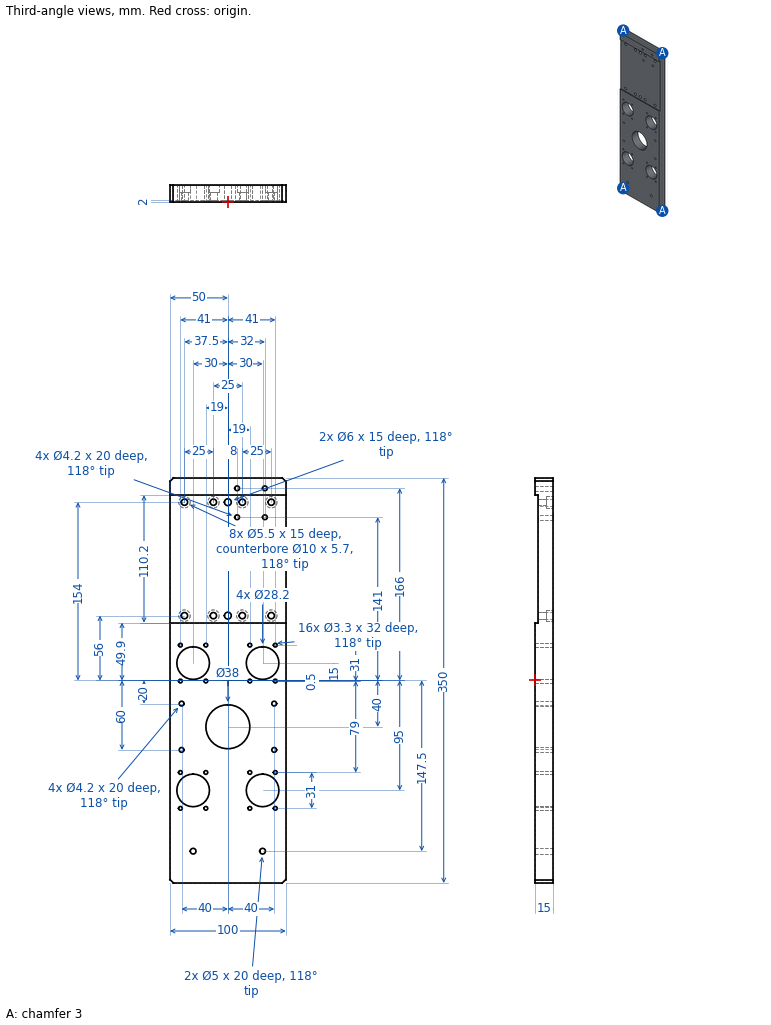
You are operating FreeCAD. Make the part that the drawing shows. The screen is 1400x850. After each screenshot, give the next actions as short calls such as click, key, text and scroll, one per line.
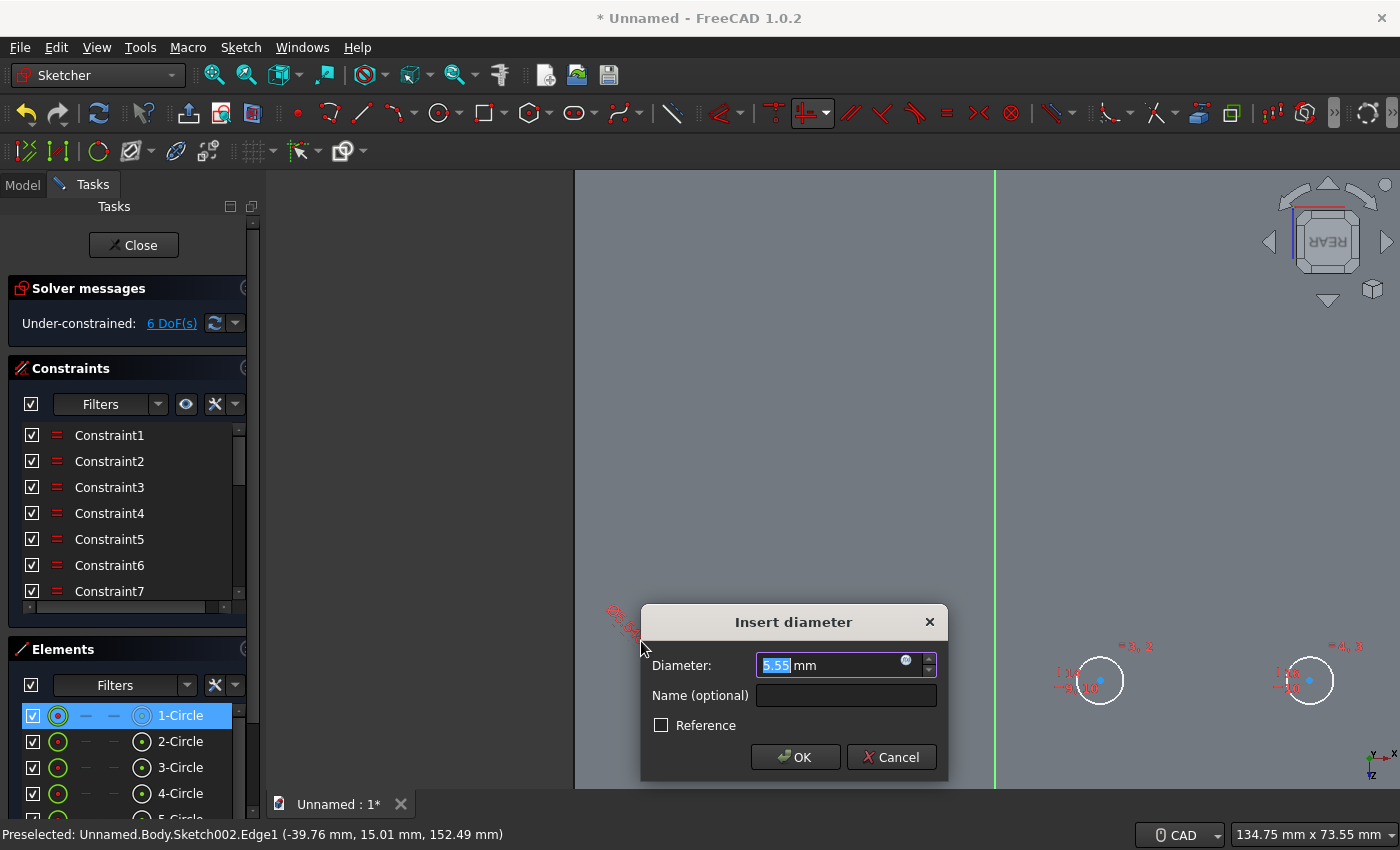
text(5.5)
key(Return)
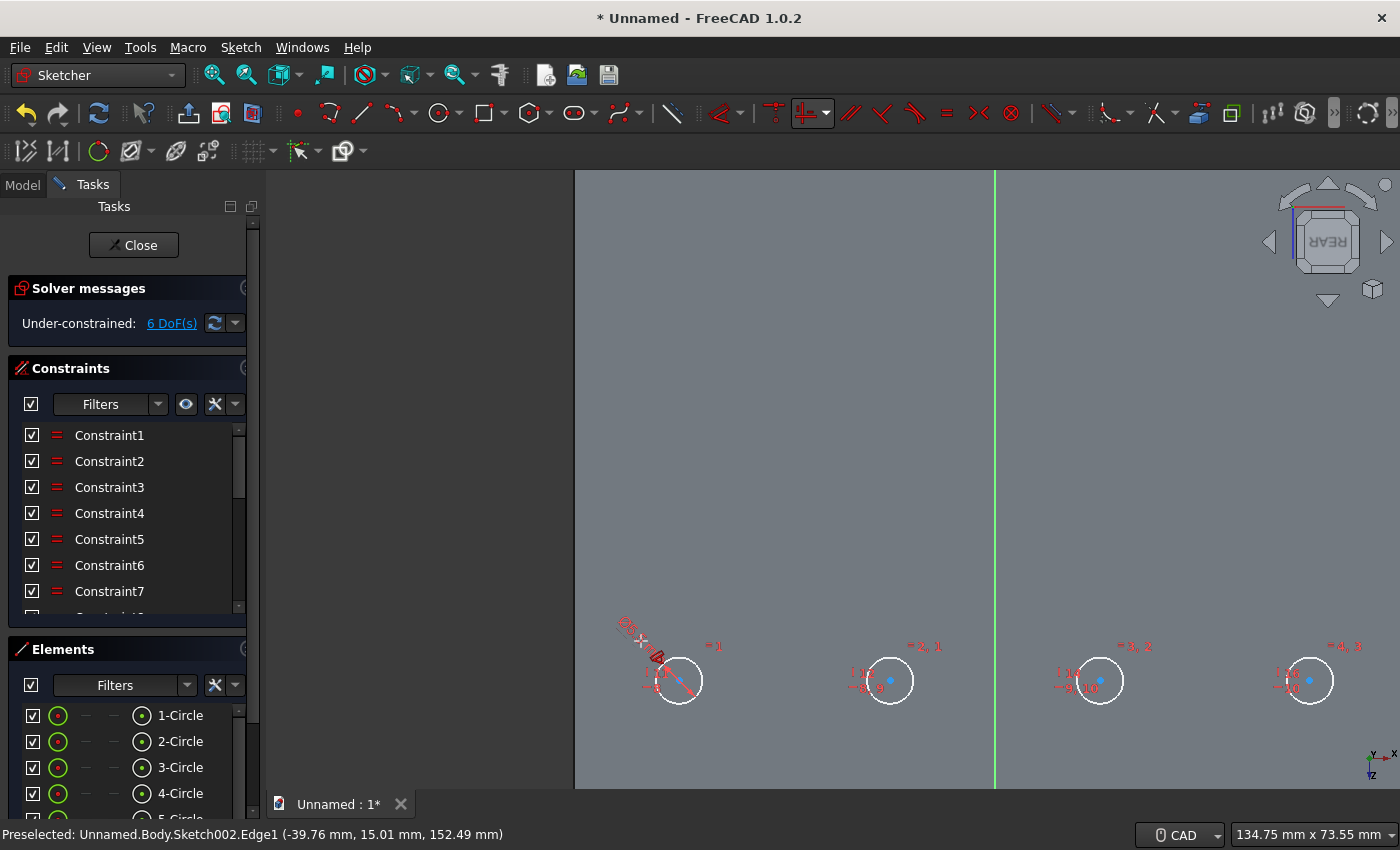
scroll(665, 668, down, 6)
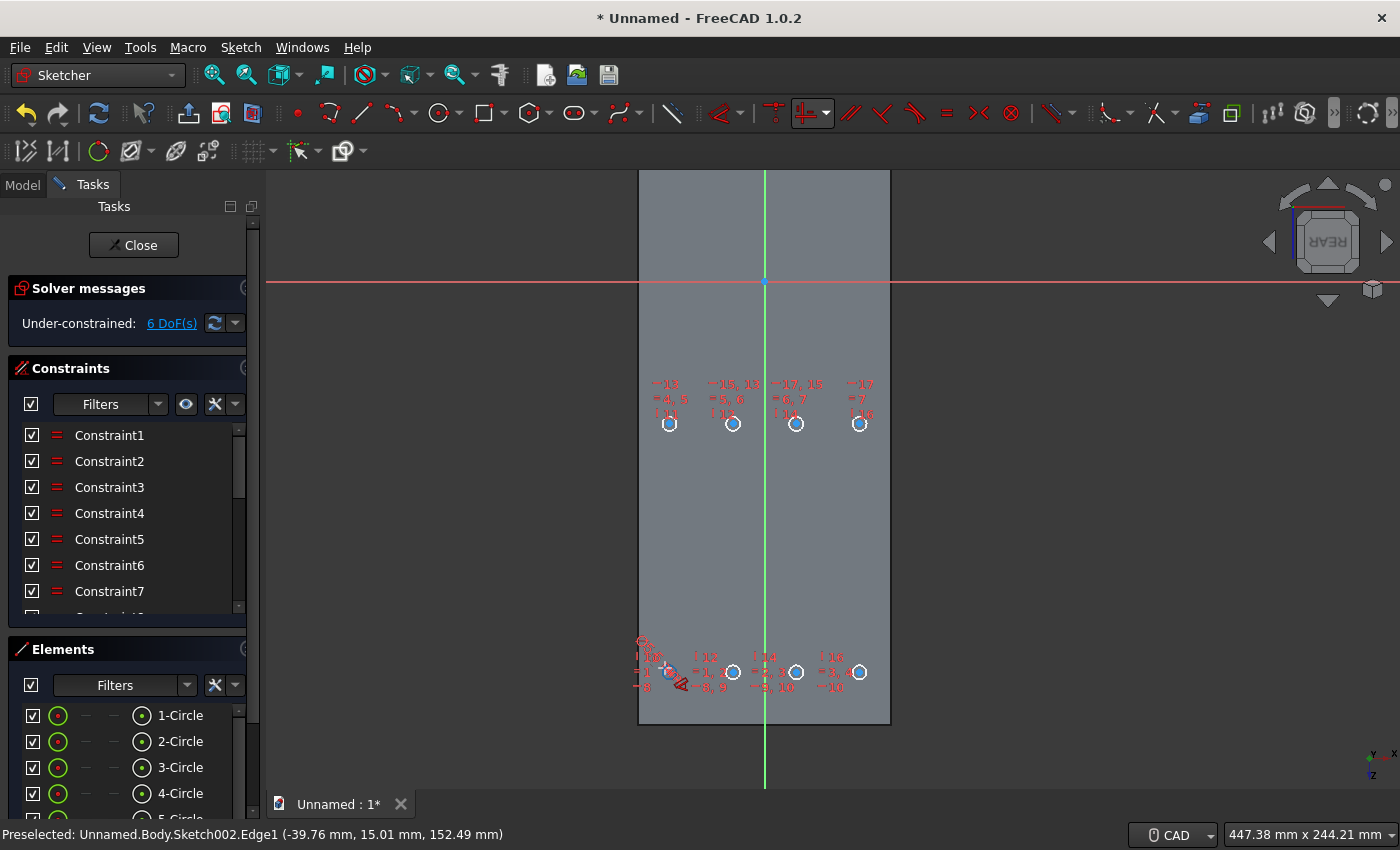
click(669, 424)
click(635, 353)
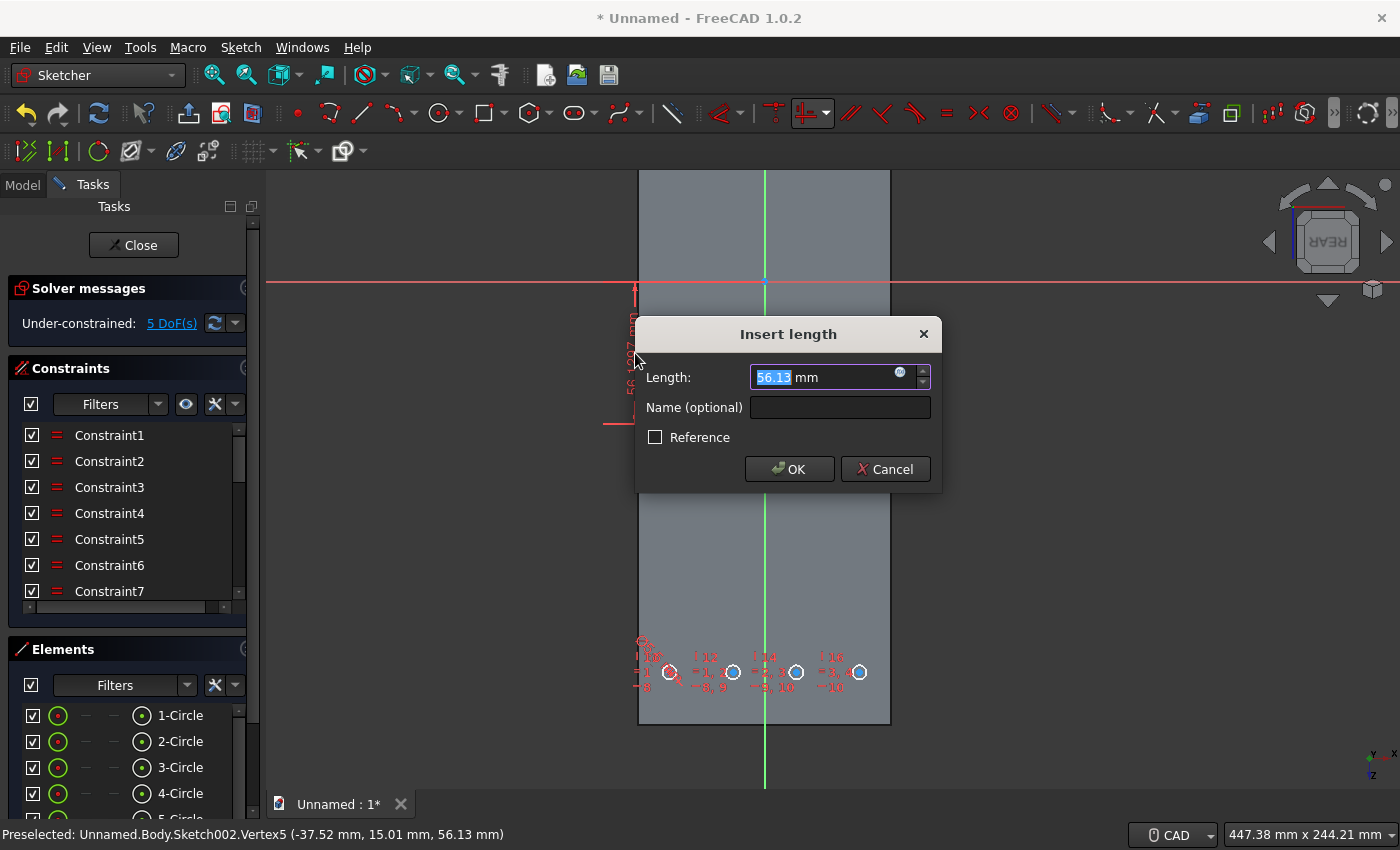
text(56)
key(Return)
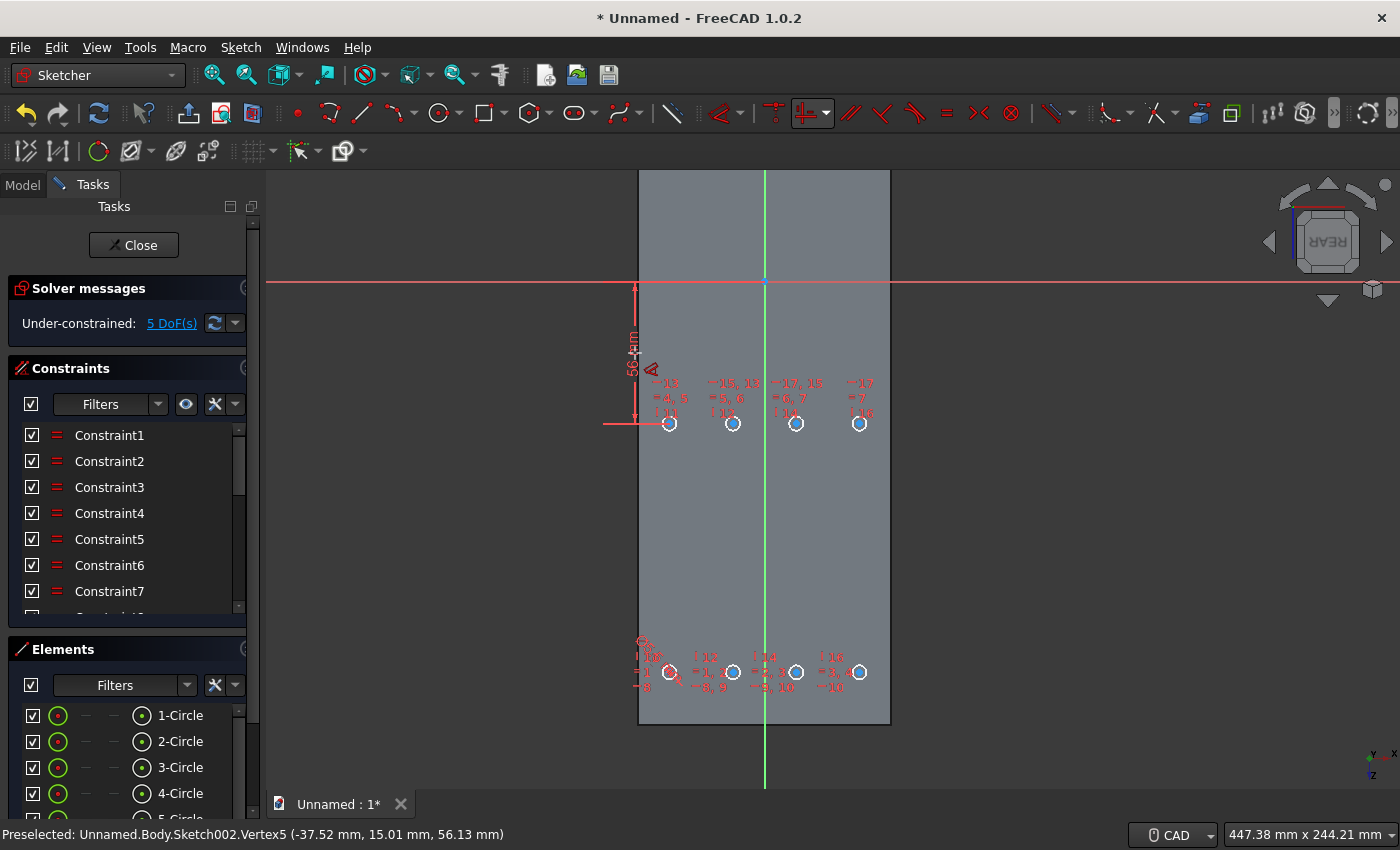
click(669, 672)
click(635, 477)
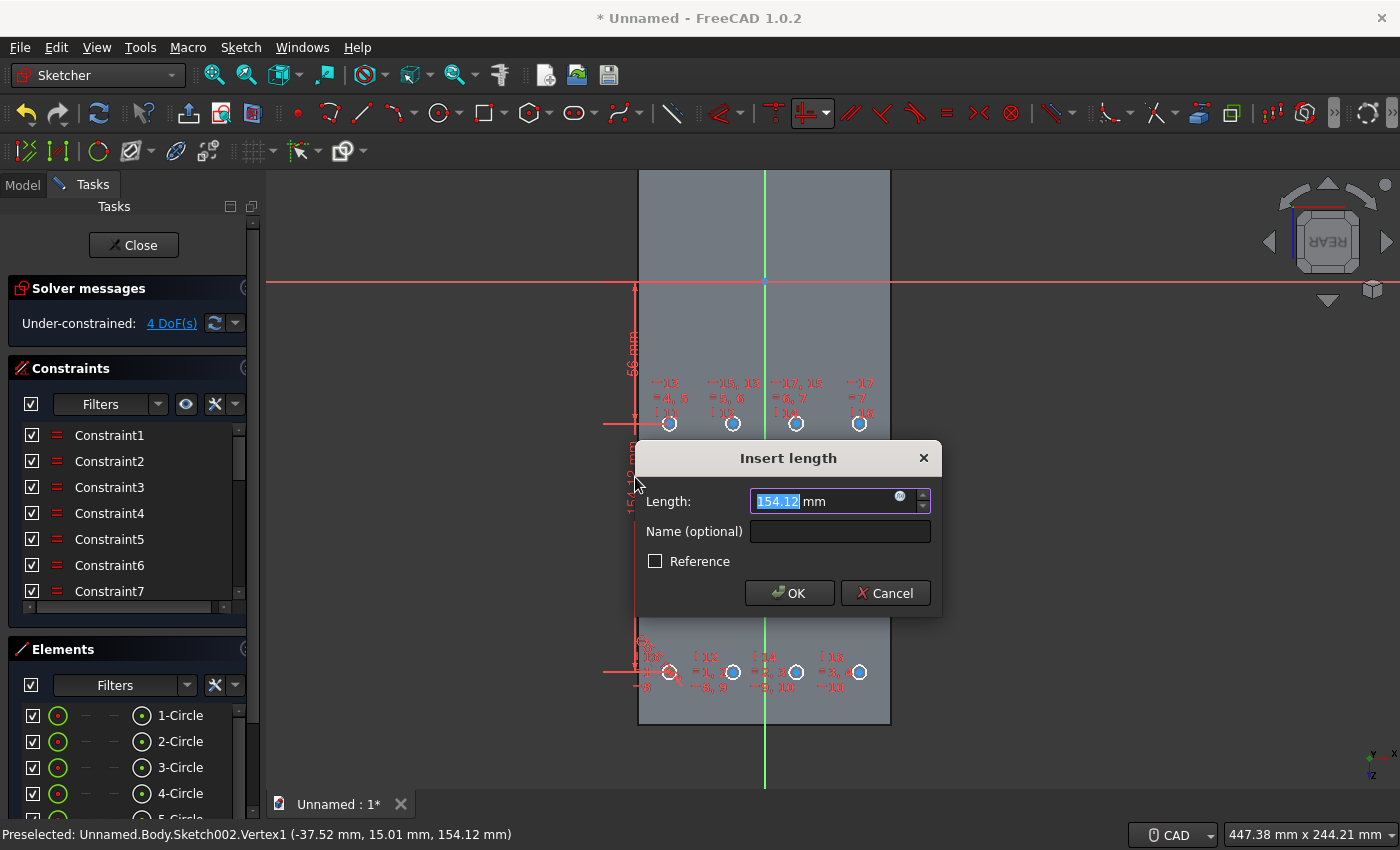
text(154)
key(Return)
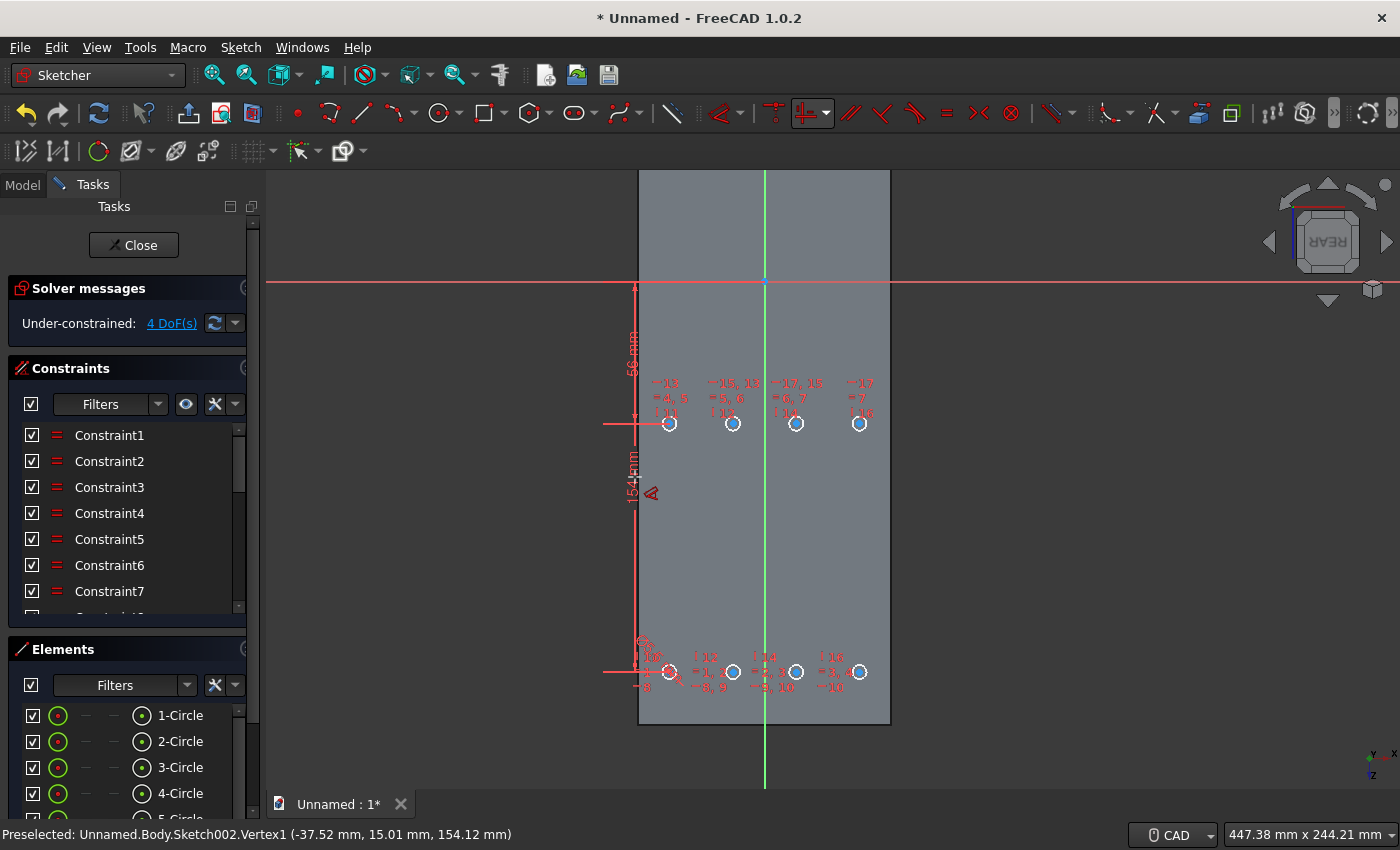
click(669, 672)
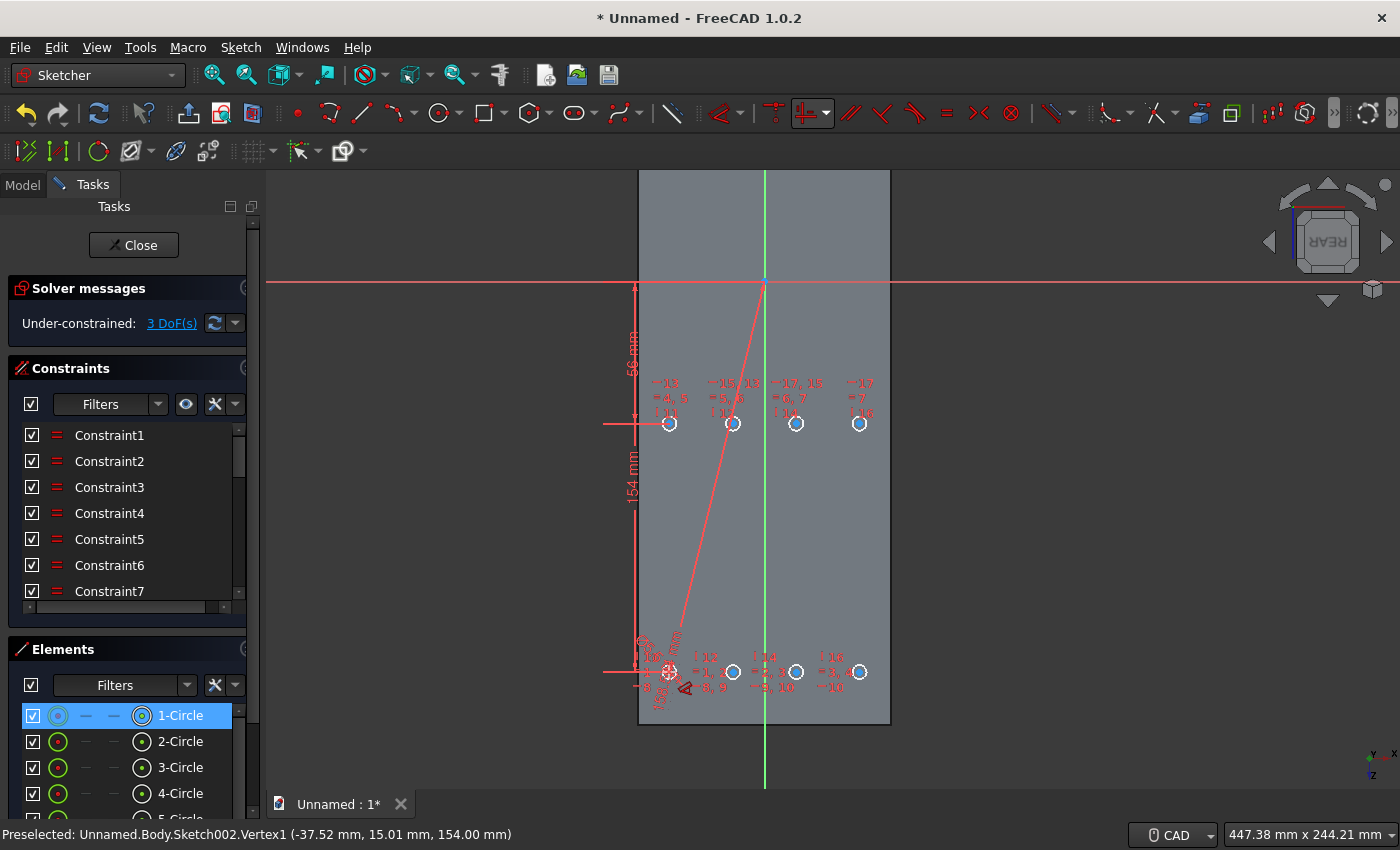
click(733, 672)
click(701, 706)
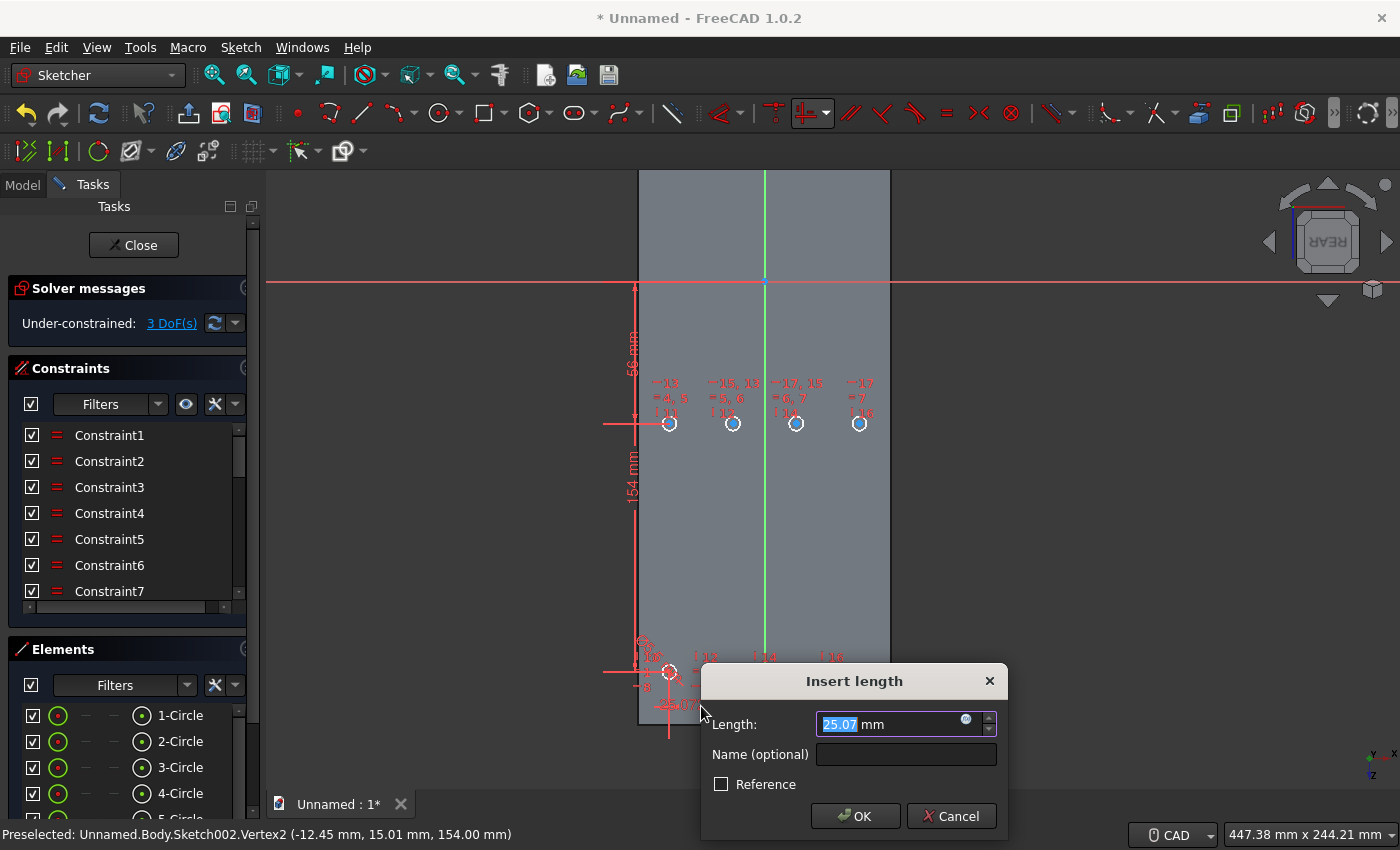
text(25)
key(Return)